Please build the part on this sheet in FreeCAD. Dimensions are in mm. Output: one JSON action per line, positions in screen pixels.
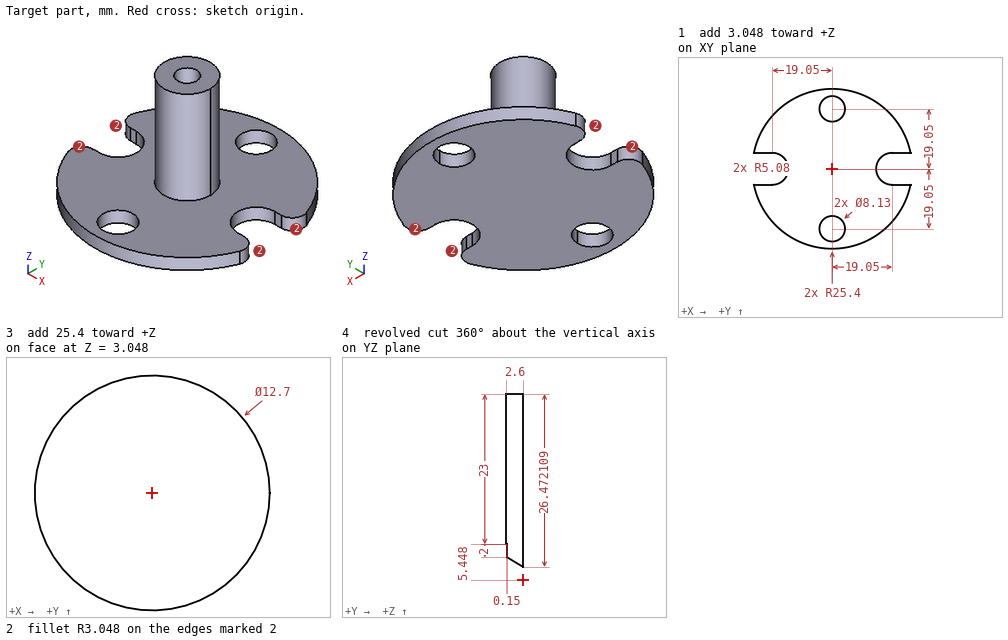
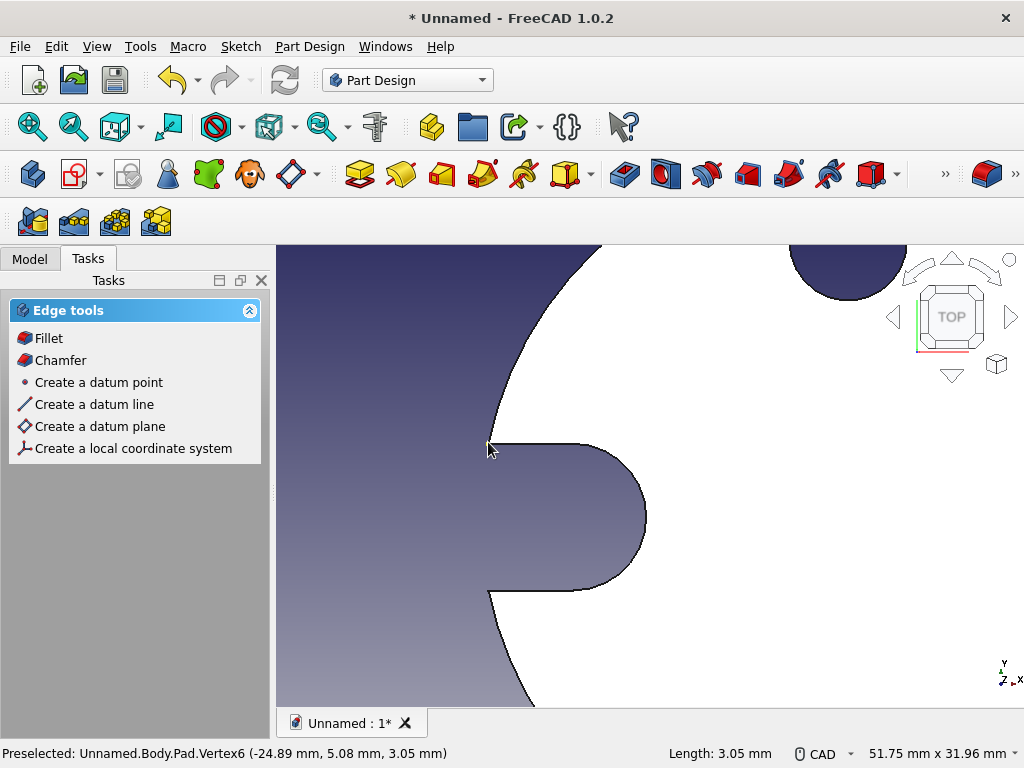
{"action": "left_click", "coordinate": [33, 128]}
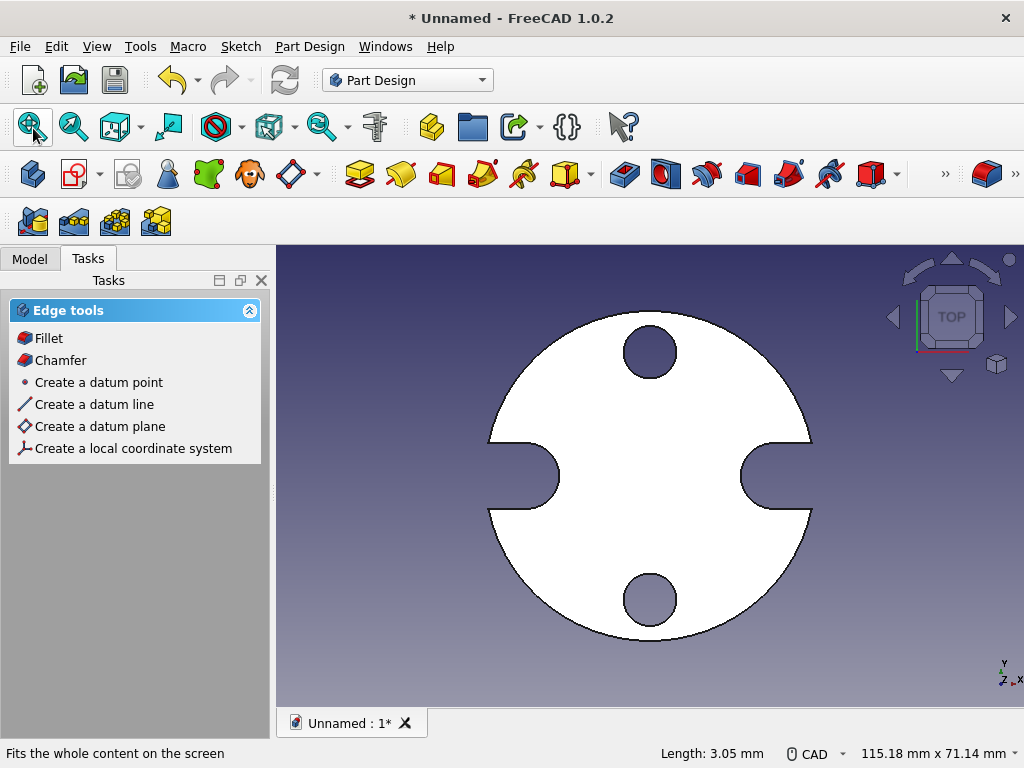
{"action": "key", "text": "1"}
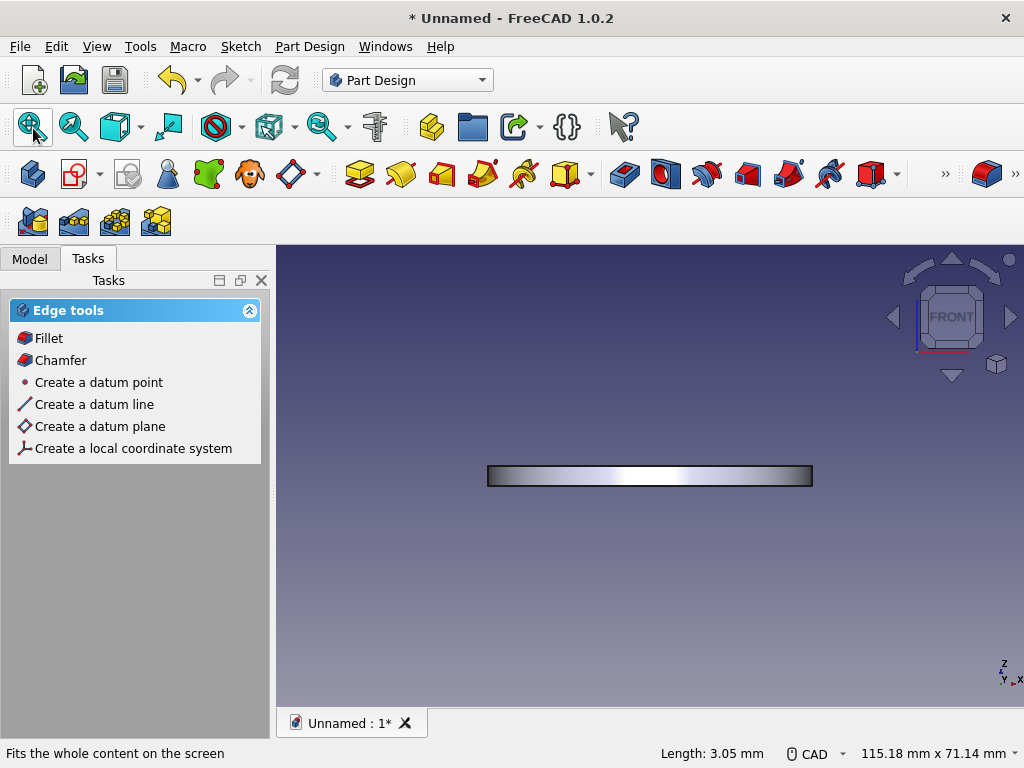
{"action": "left_click", "coordinate": [33, 128]}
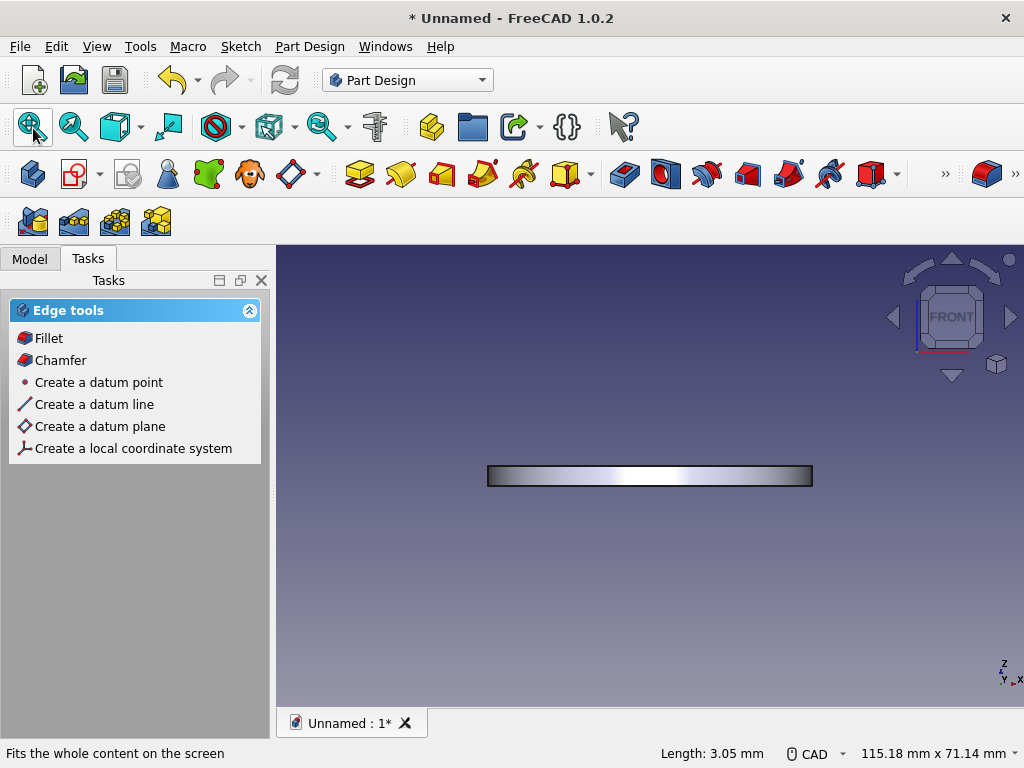
{"action": "scroll", "coordinate": [488, 475], "scroll_direction": "up", "scroll_amount": 4}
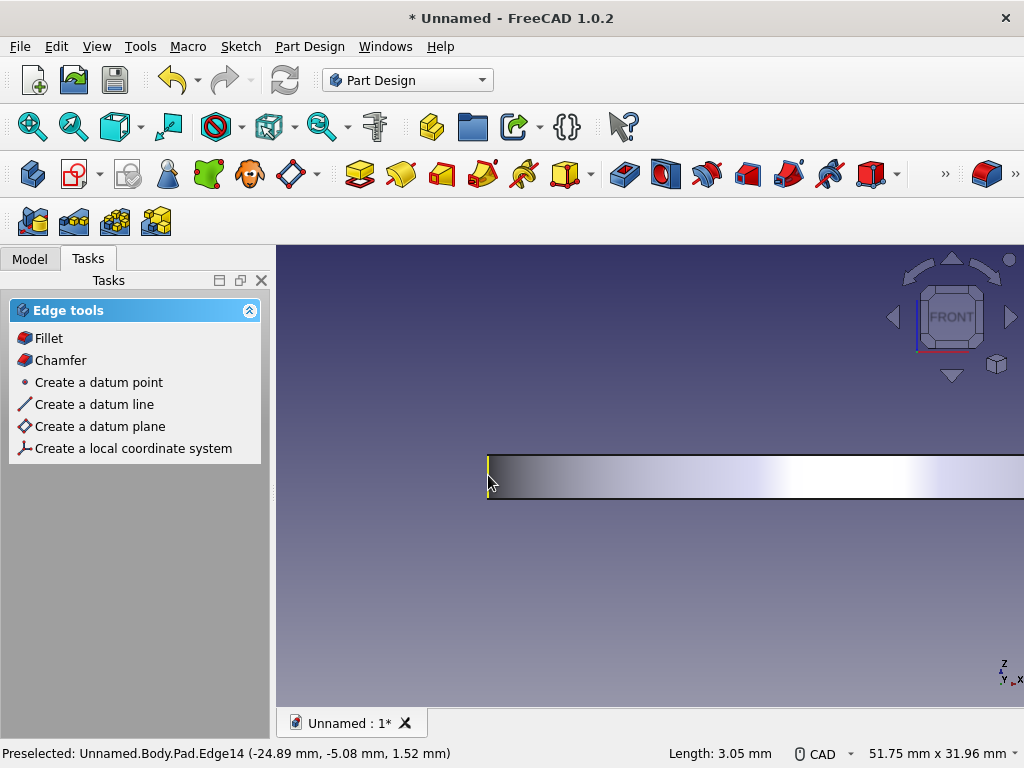
{"action": "left_click", "coordinate": [33, 128]}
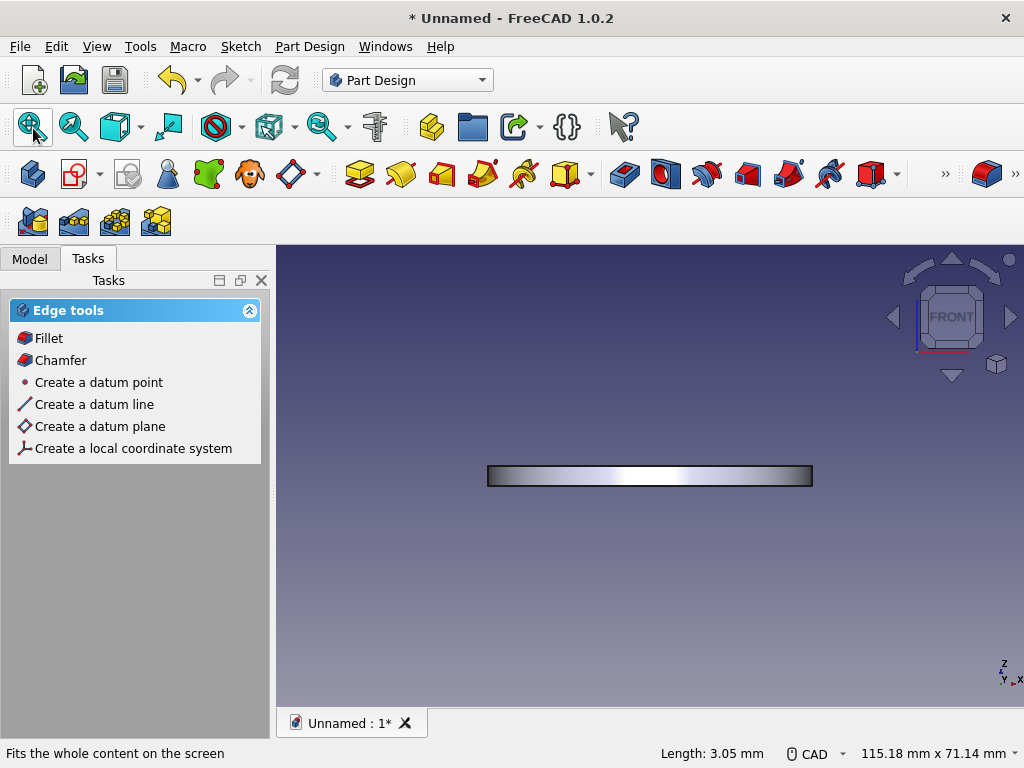
{"action": "key", "text": "3"}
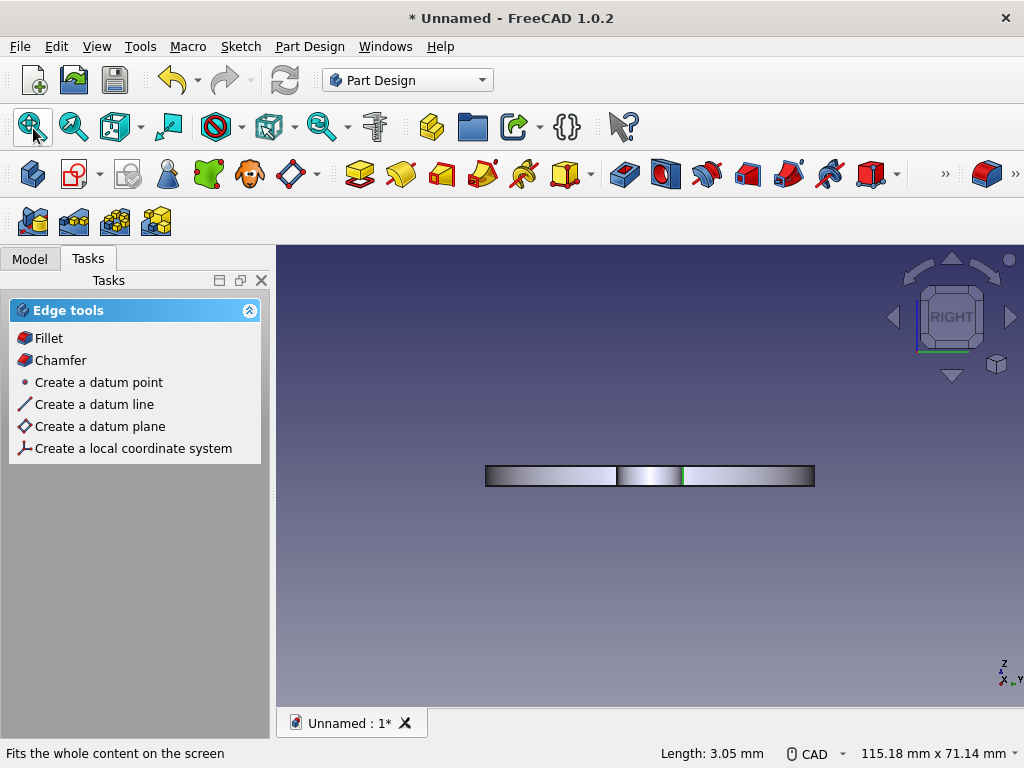
{"action": "left_click", "coordinate": [33, 128]}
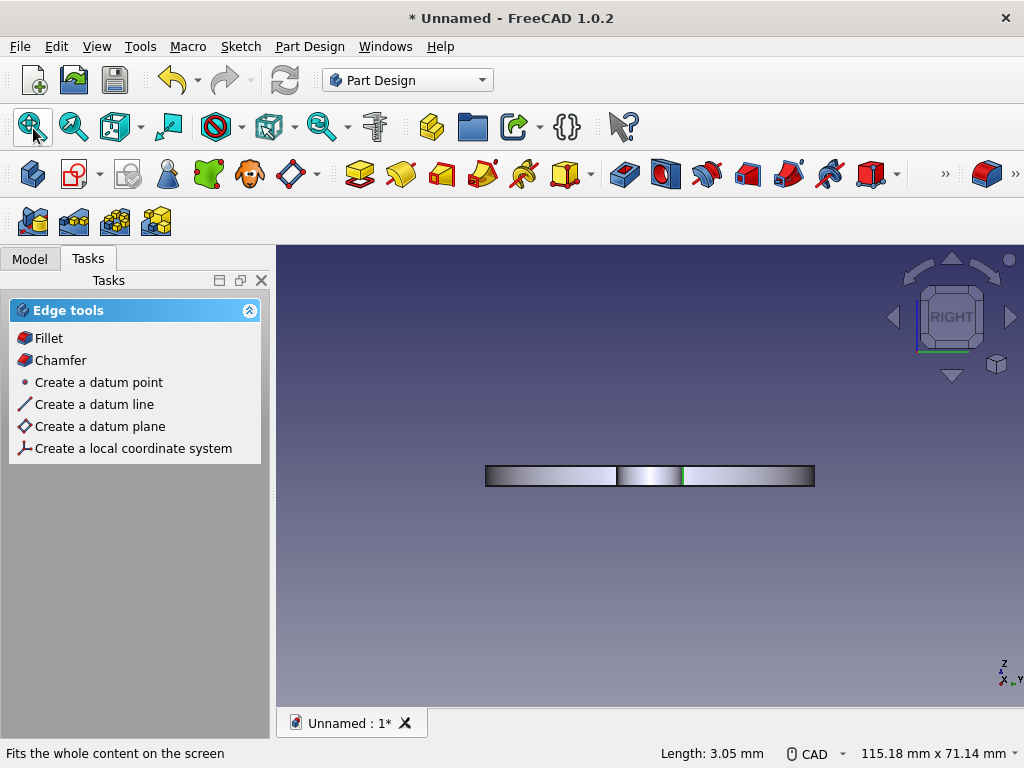
{"action": "left_click", "coordinate": [617, 475], "text": "ctrl"}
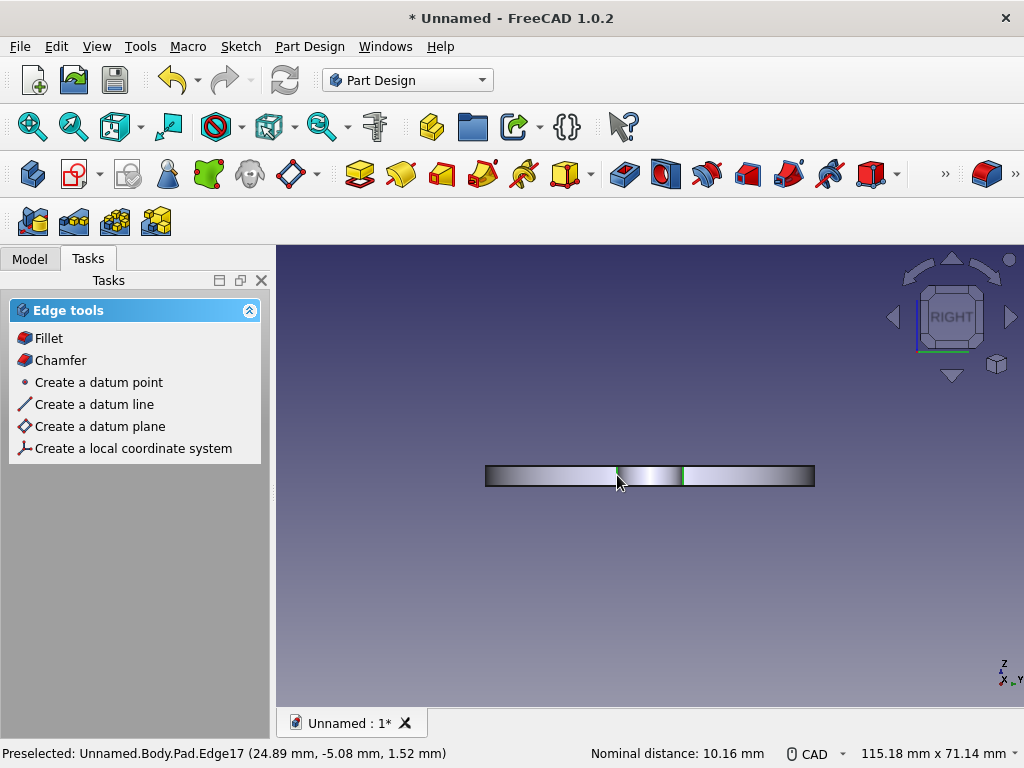
{"action": "scroll", "coordinate": [683, 475], "scroll_direction": "up", "scroll_amount": 4}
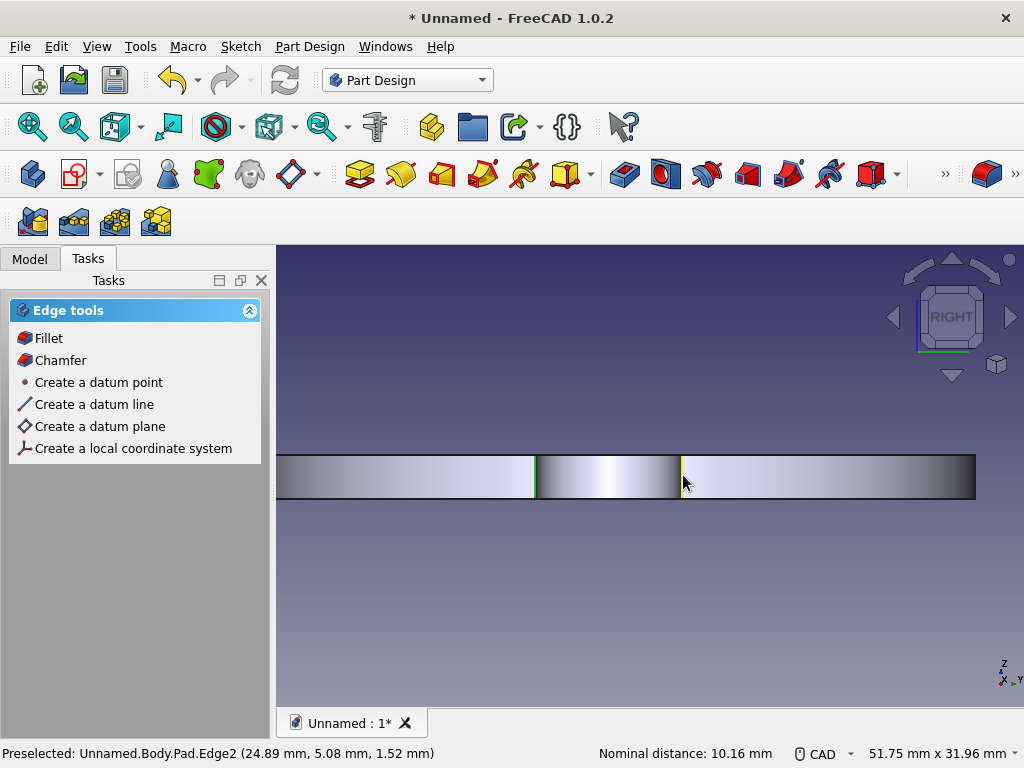
{"action": "left_click", "coordinate": [33, 128]}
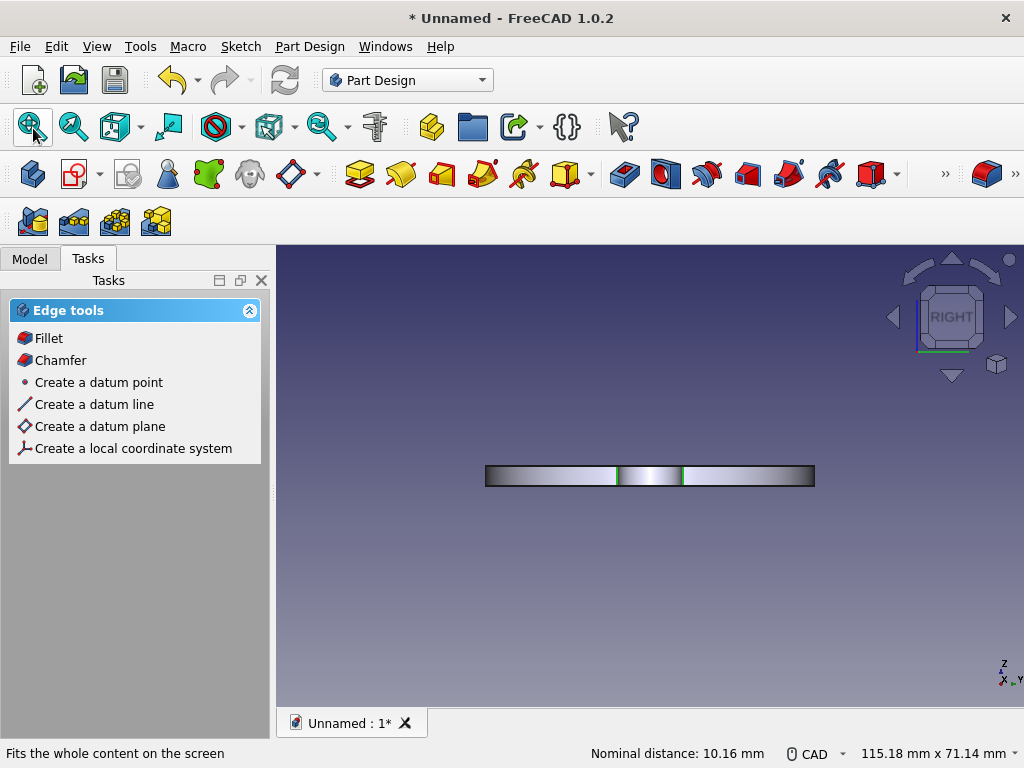
{"action": "key", "text": "5"}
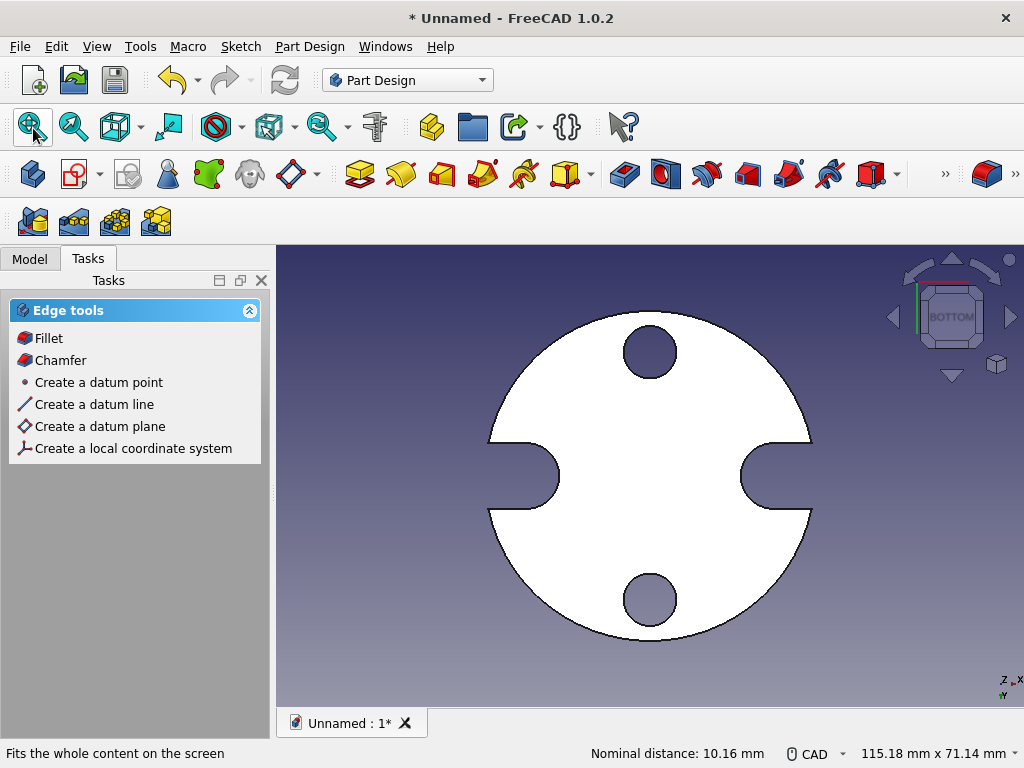
{"action": "scroll", "coordinate": [488, 508], "scroll_direction": "up", "scroll_amount": 4}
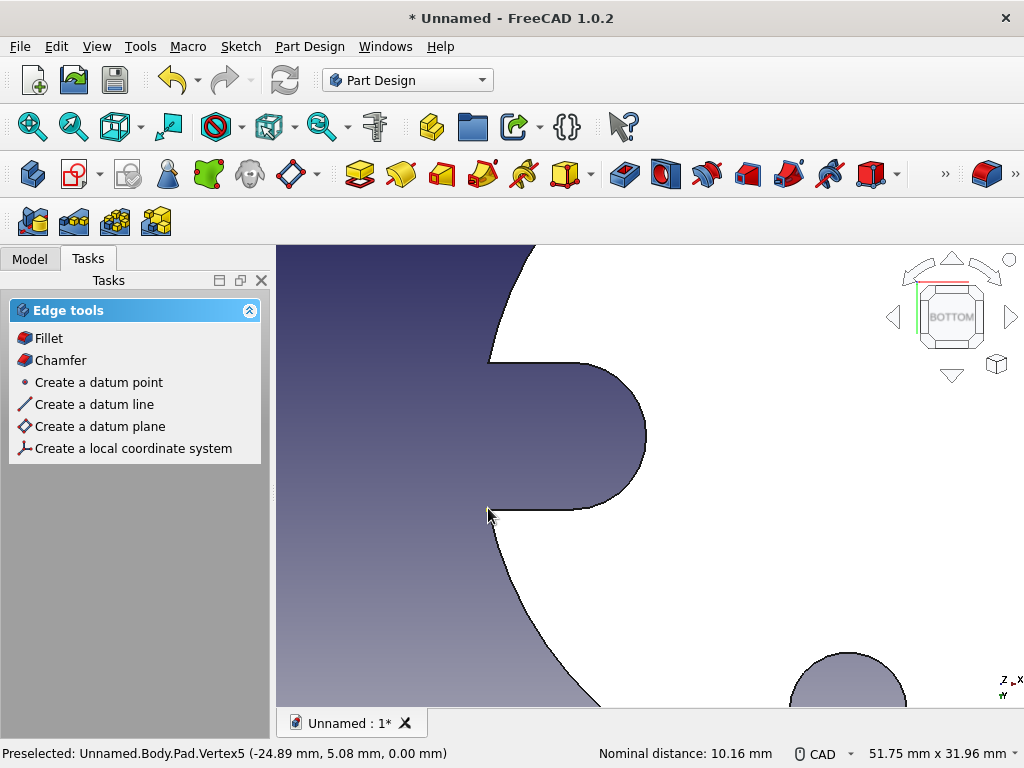
{"action": "left_click", "coordinate": [33, 128]}